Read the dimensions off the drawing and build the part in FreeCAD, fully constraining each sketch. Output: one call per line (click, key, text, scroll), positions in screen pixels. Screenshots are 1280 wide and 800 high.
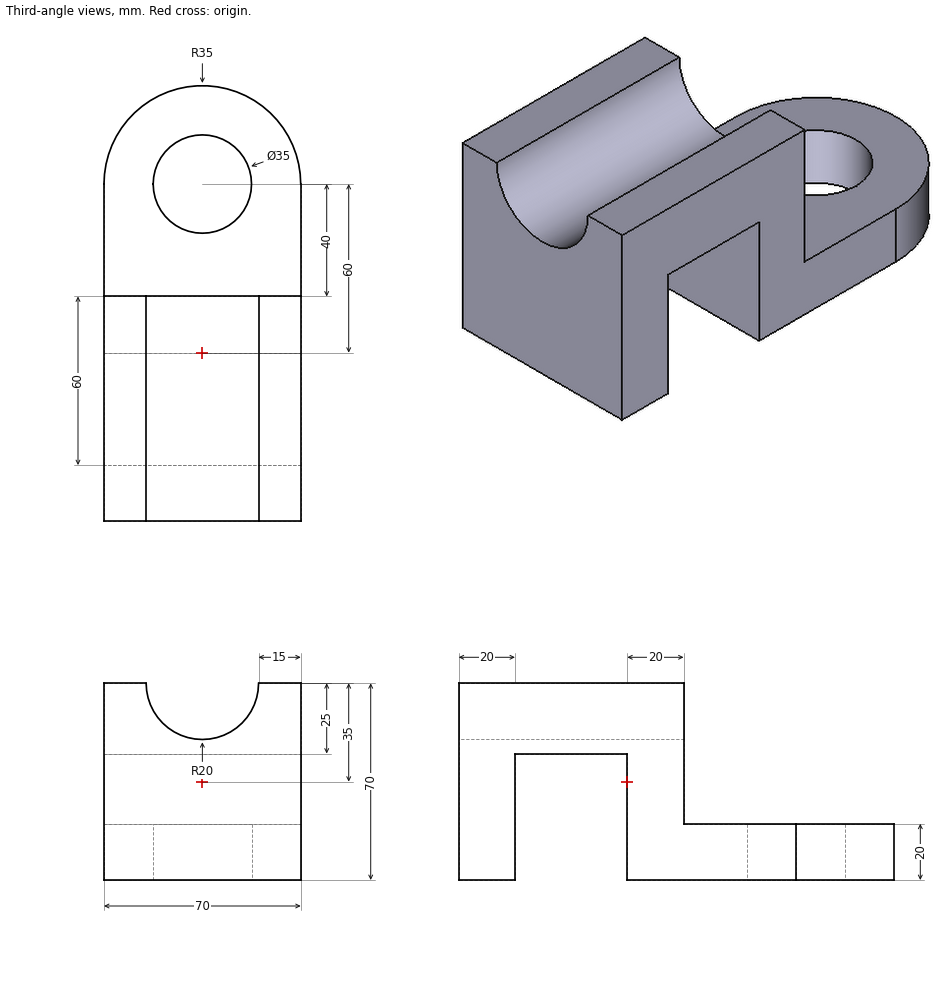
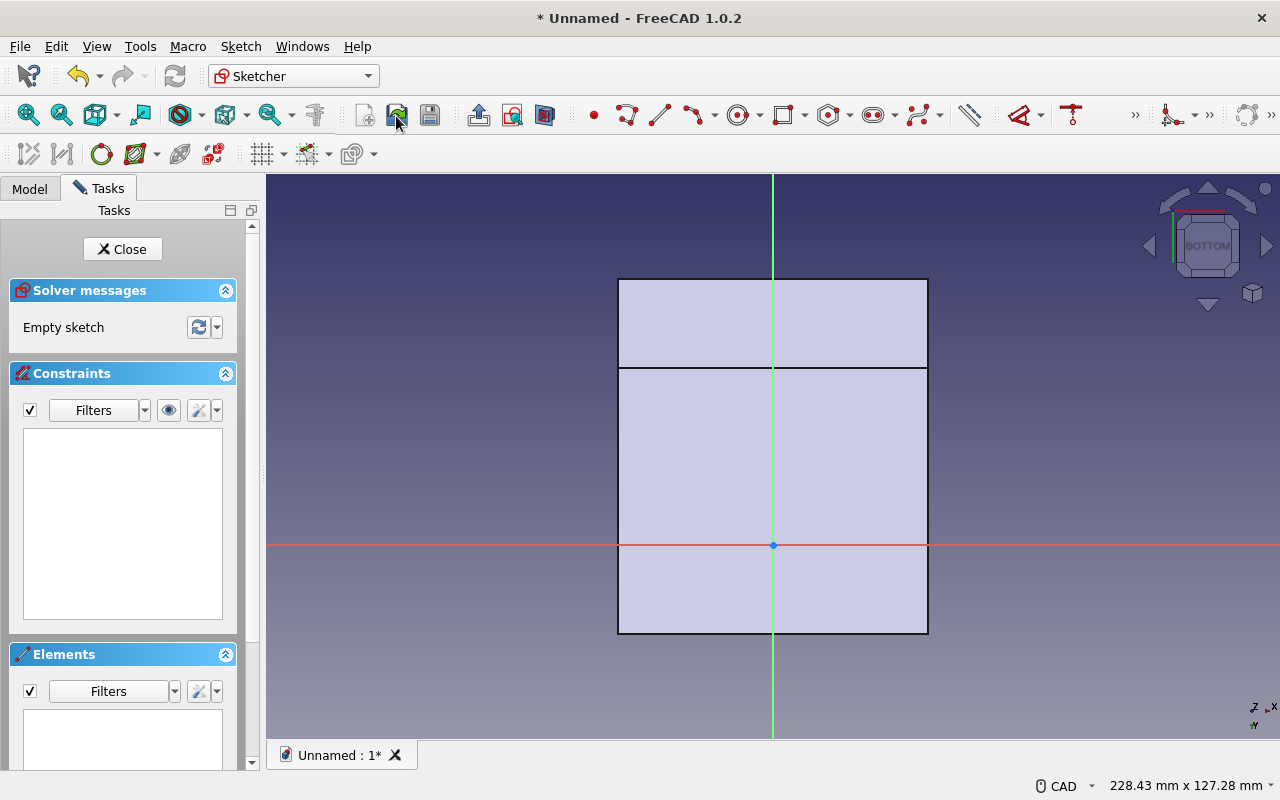
scroll(621, 202, down, 3)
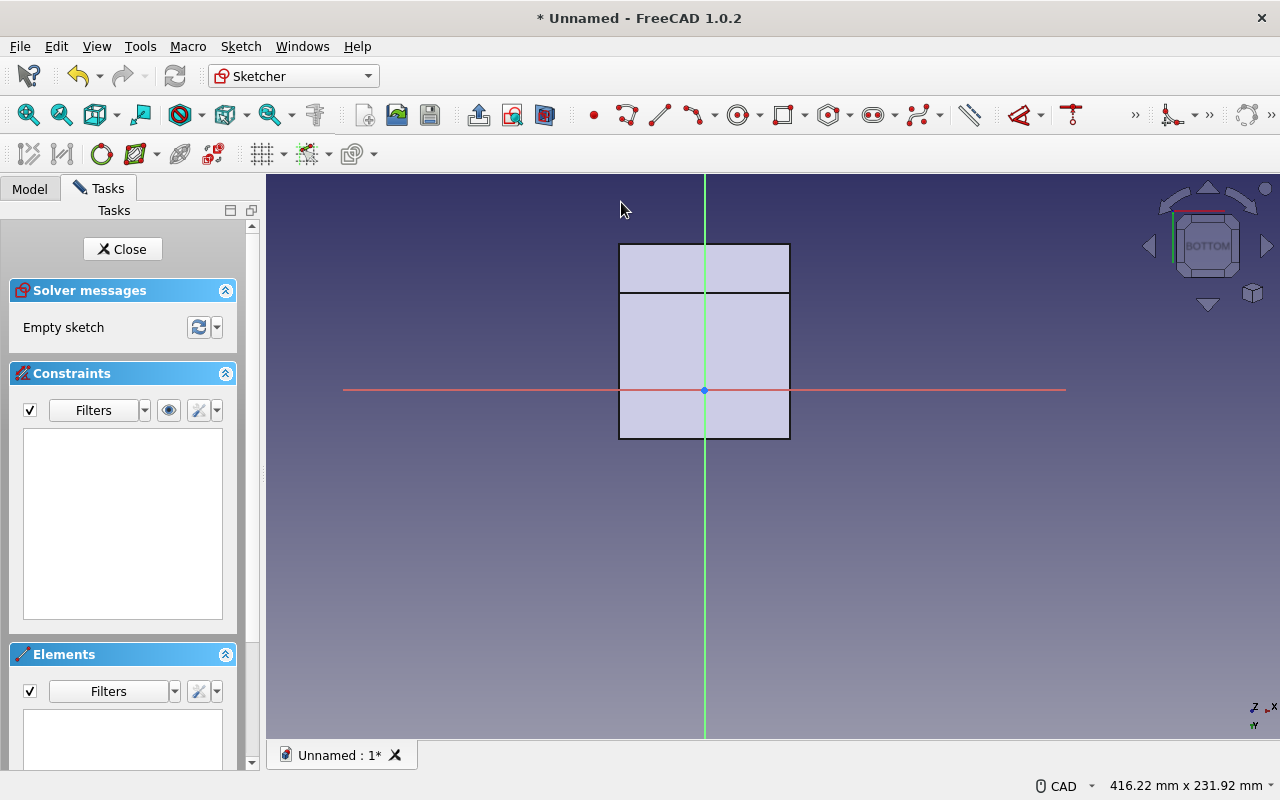
scroll(705, 607, up, 2)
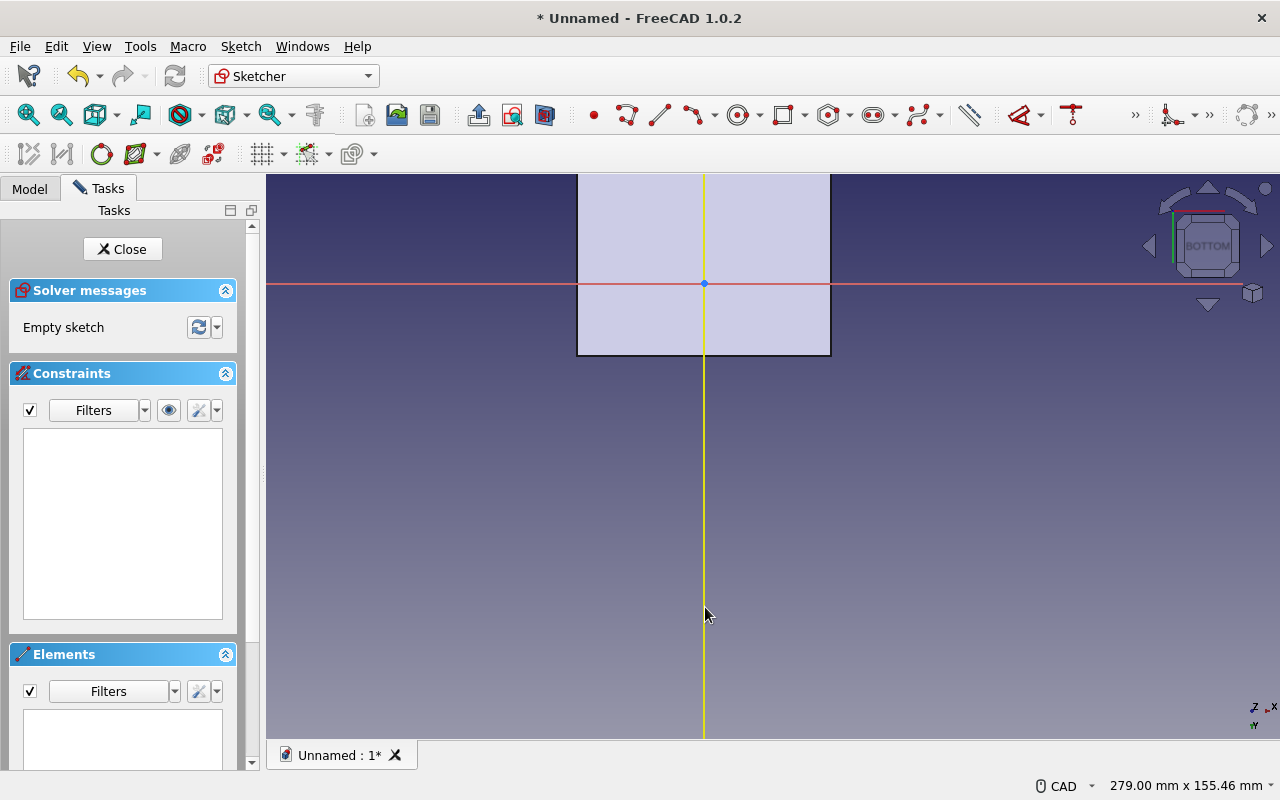
click(627, 116)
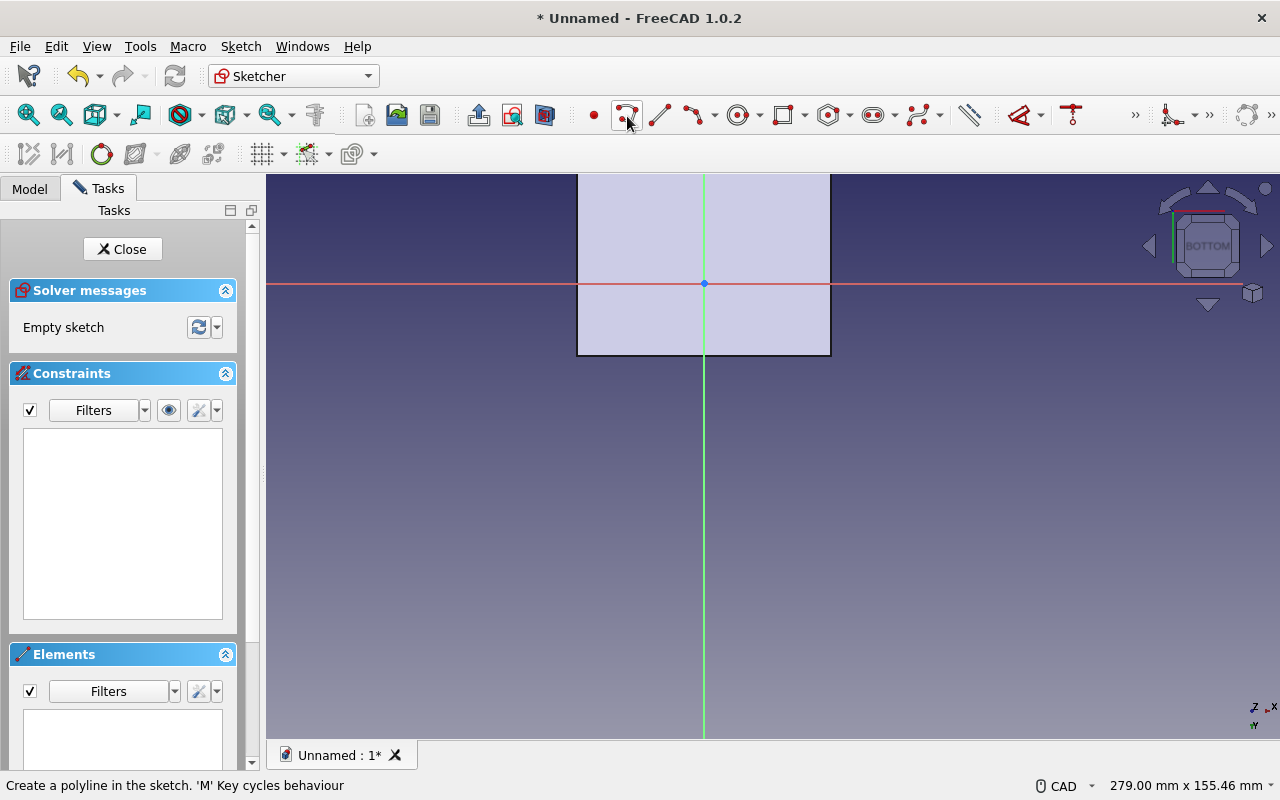
click(831, 502)
click(831, 356)
click(577, 356)
click(577, 502)
right_click(577, 502)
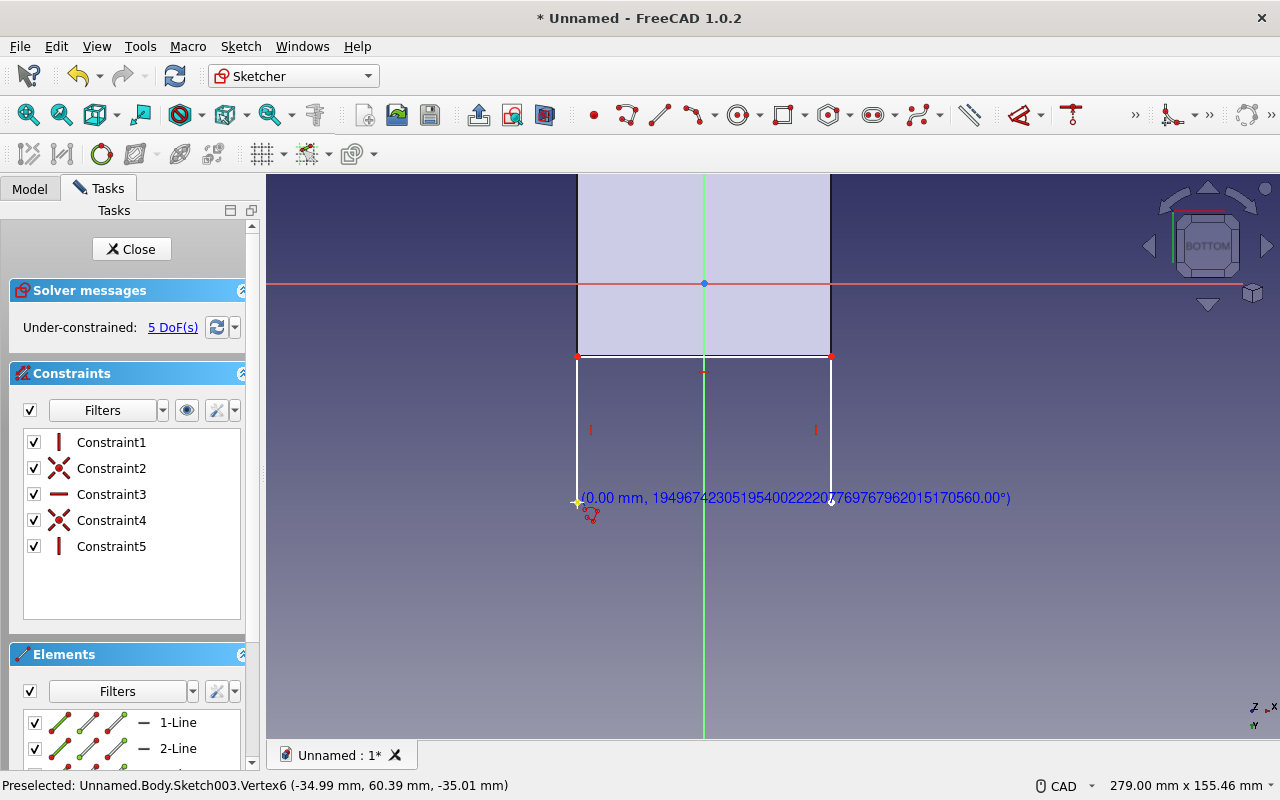
click(692, 116)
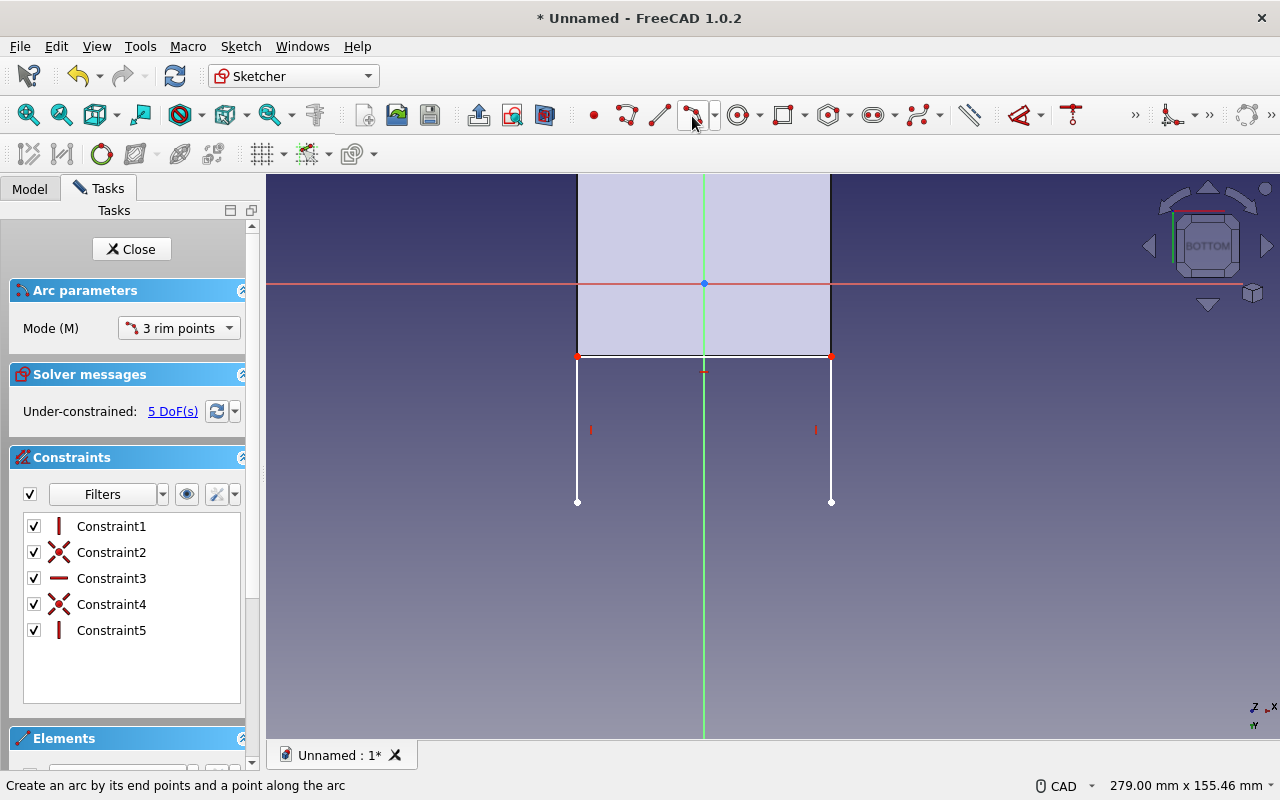
click(577, 503)
click(831, 503)
click(665, 623)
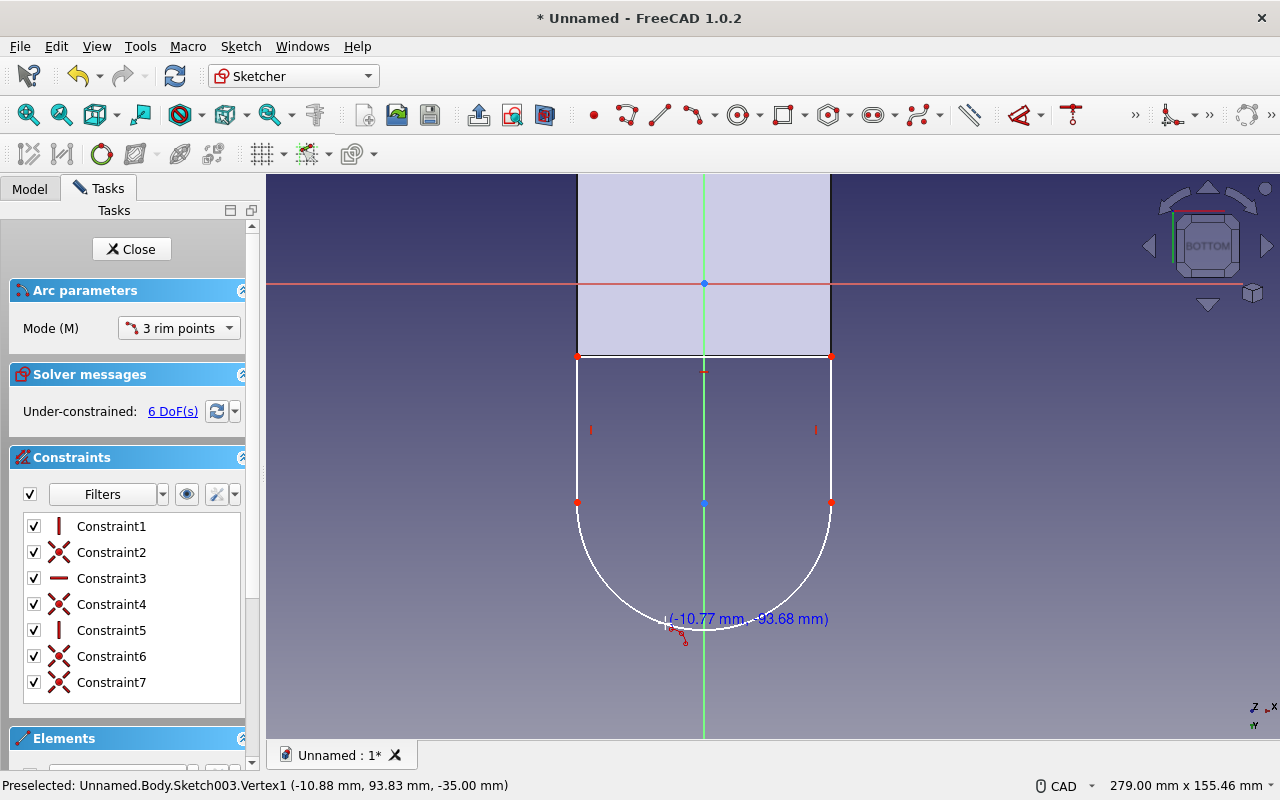
click(738, 116)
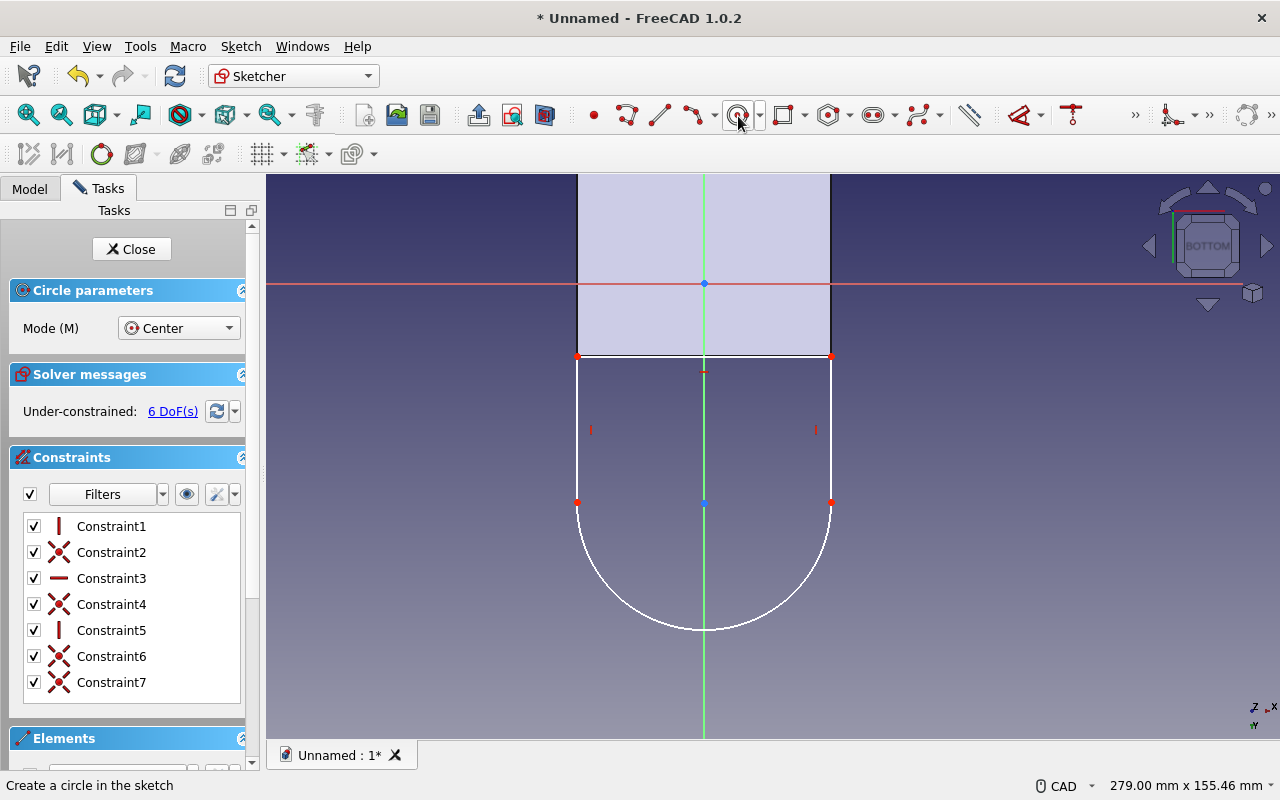
click(704, 502)
click(749, 457)
key(Escape)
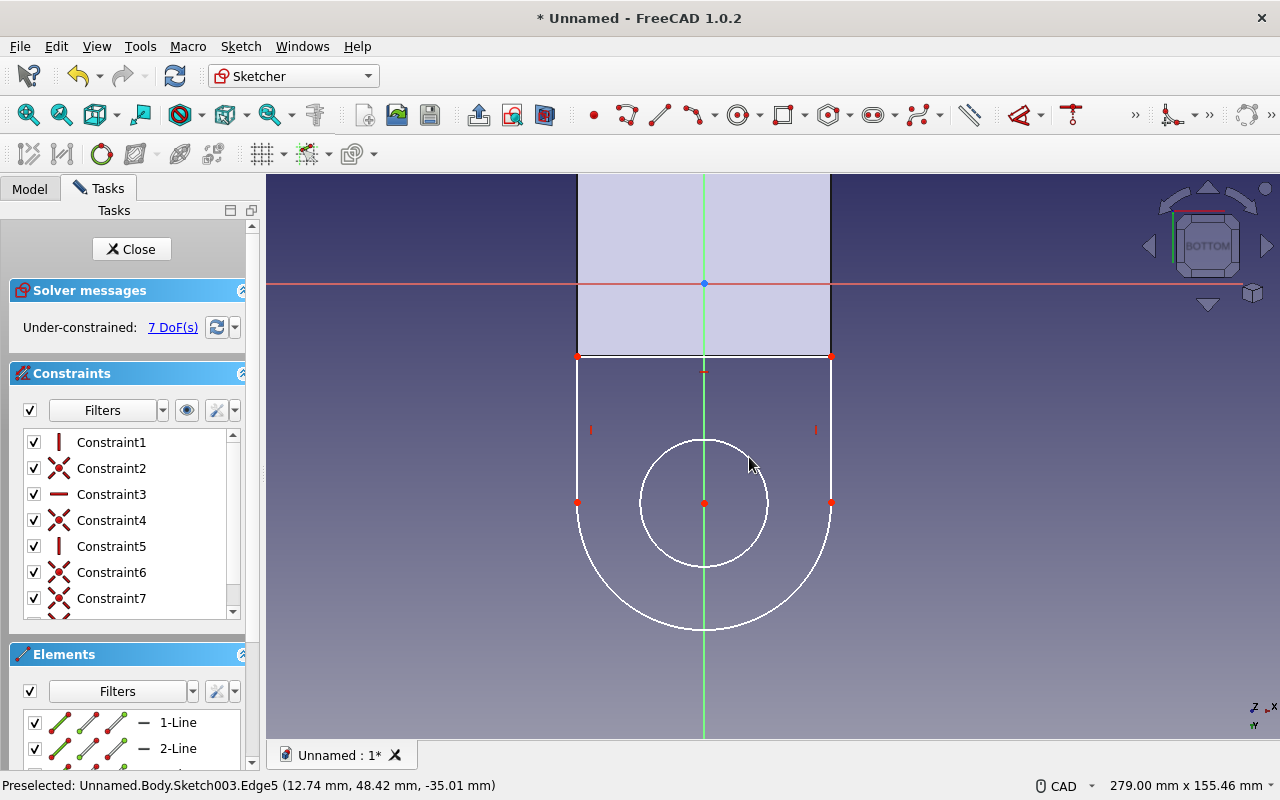
click(831, 459)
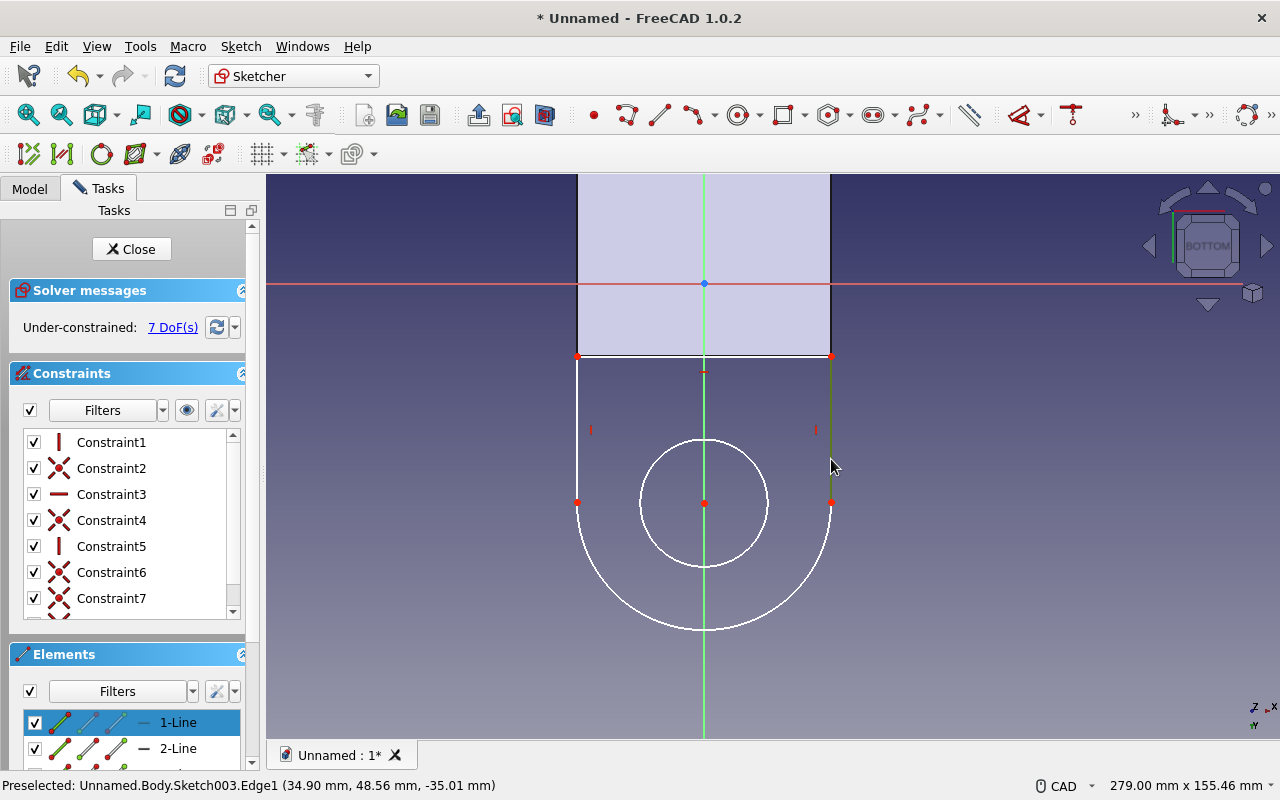
click(629, 606)